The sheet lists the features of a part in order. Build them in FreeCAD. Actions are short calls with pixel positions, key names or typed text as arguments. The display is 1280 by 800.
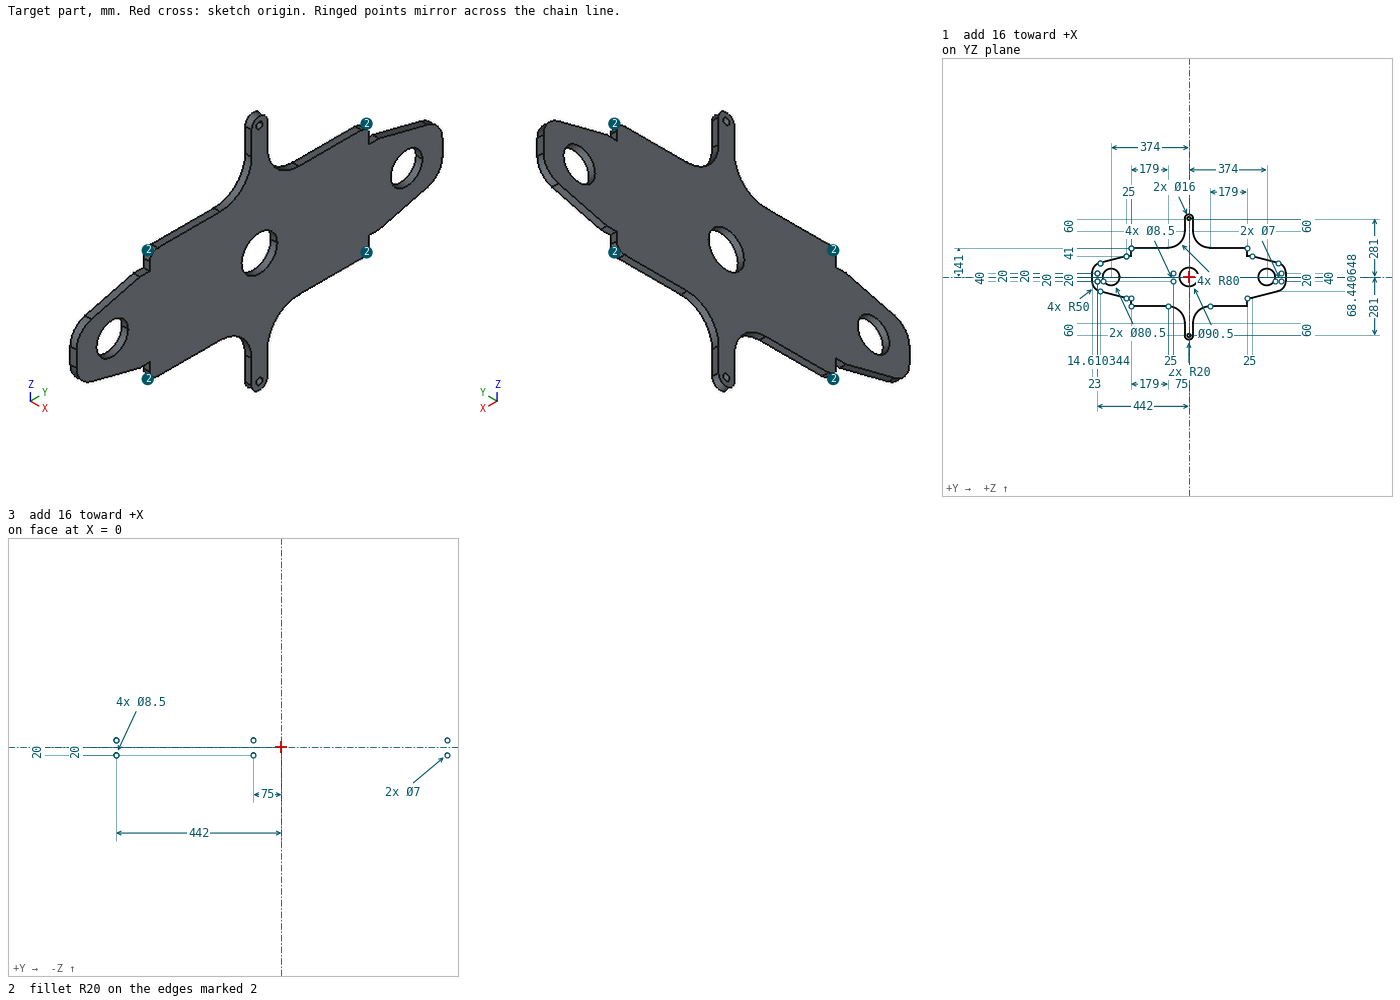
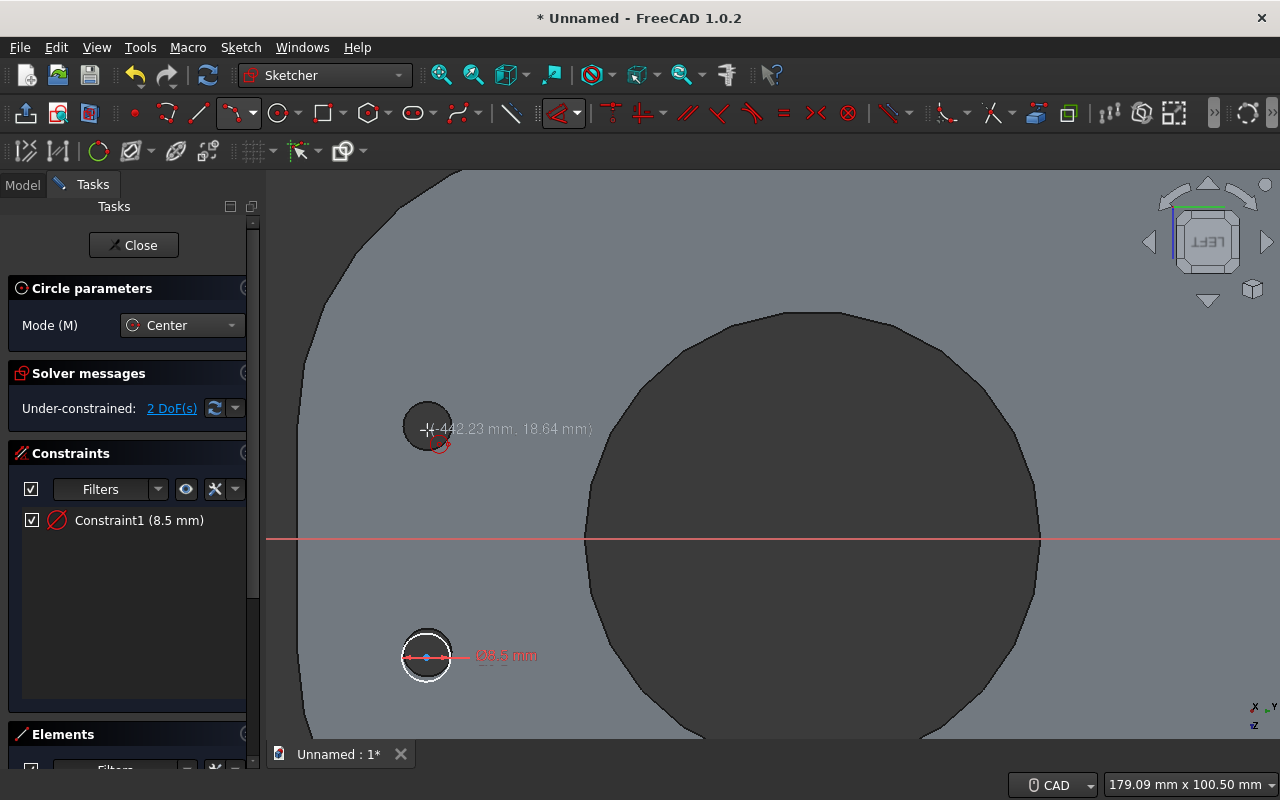
scroll(427, 444, down, 11)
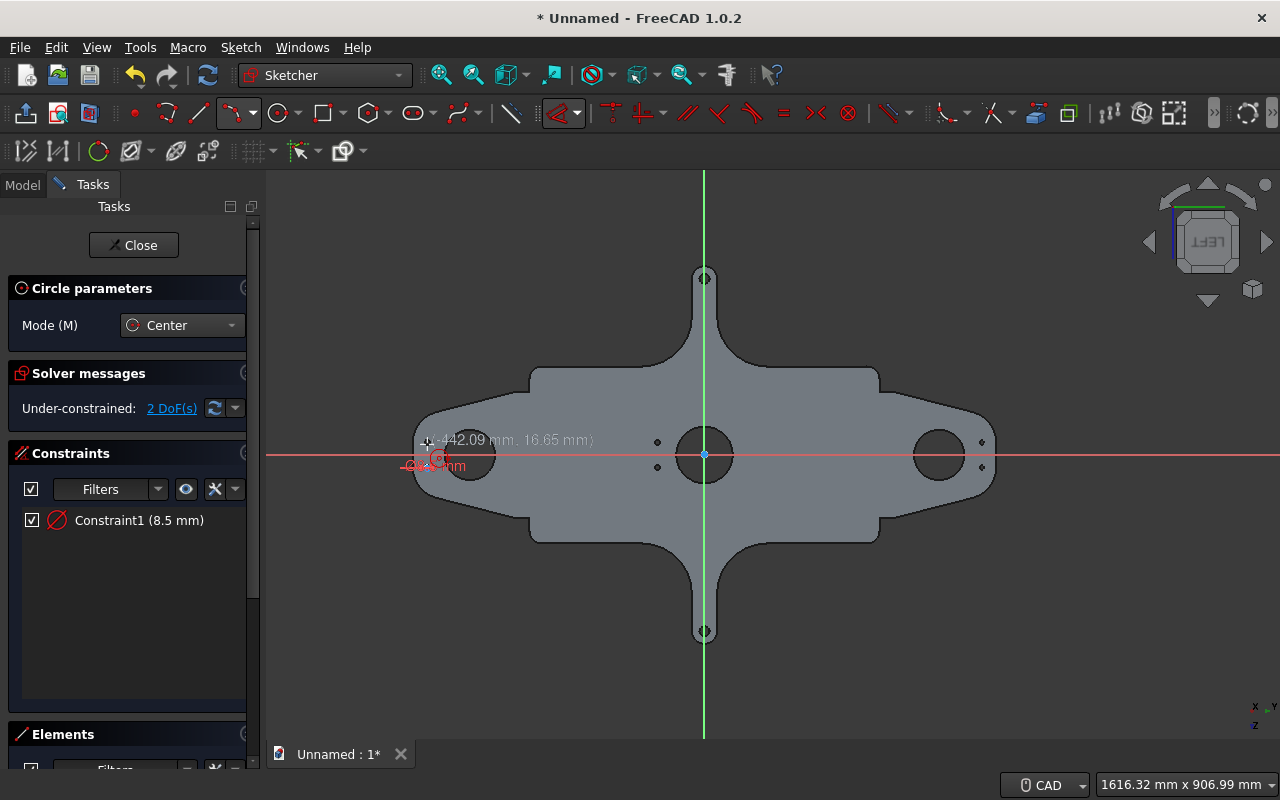
scroll(427, 442, up, 2)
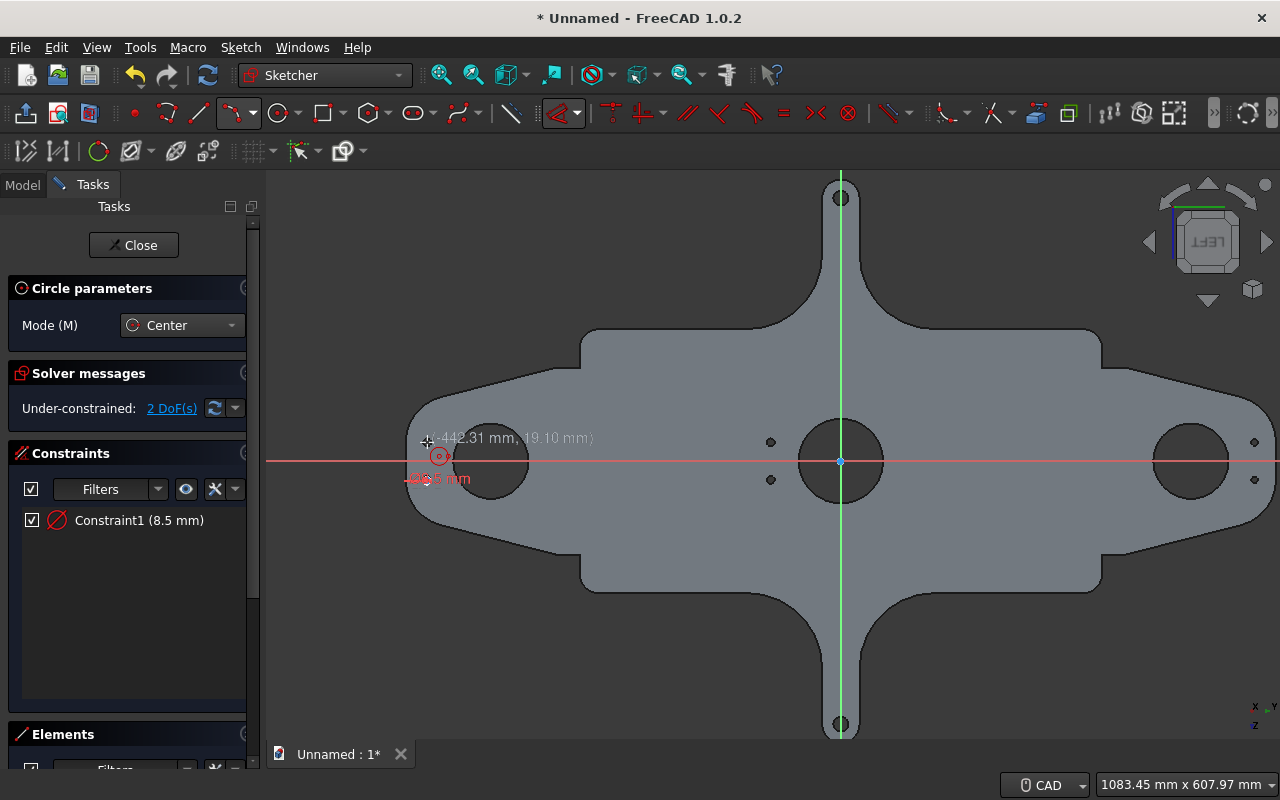
click(427, 442)
move(430, 440)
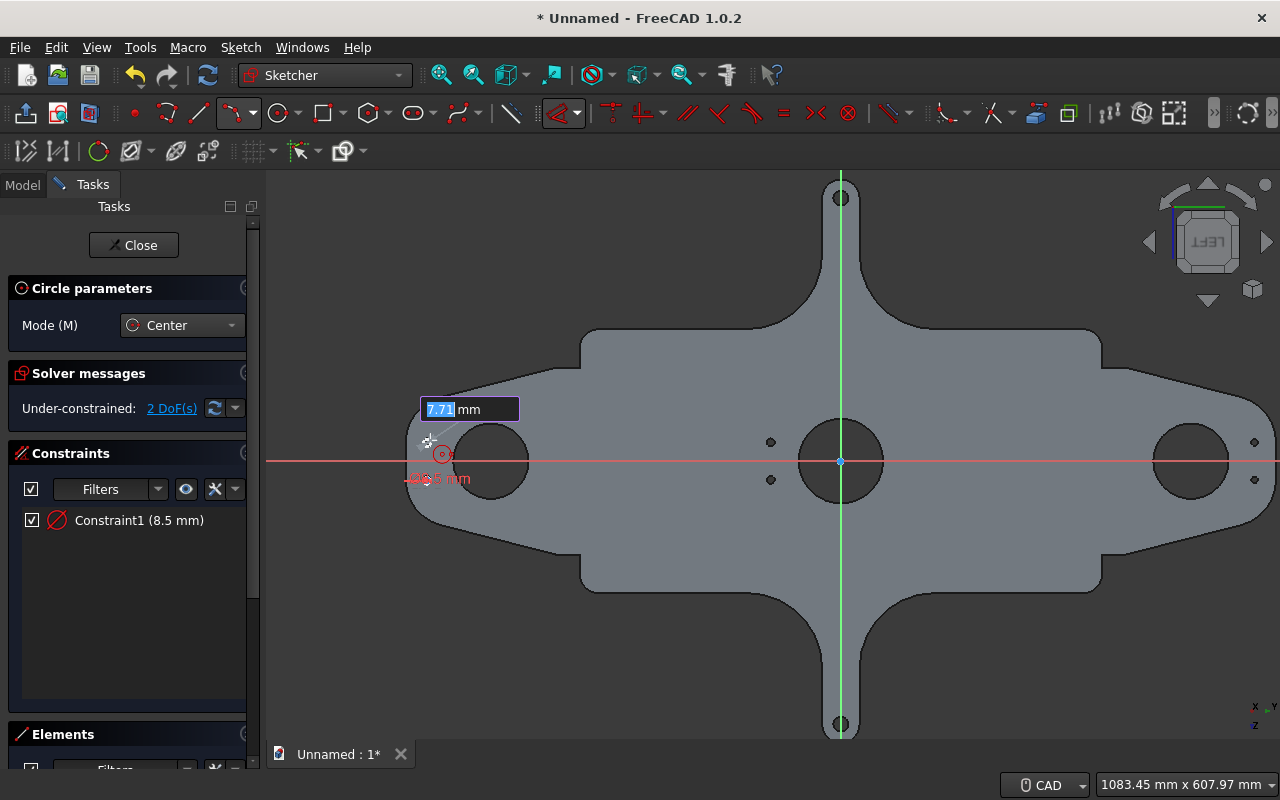
text(8.5)
key(Return)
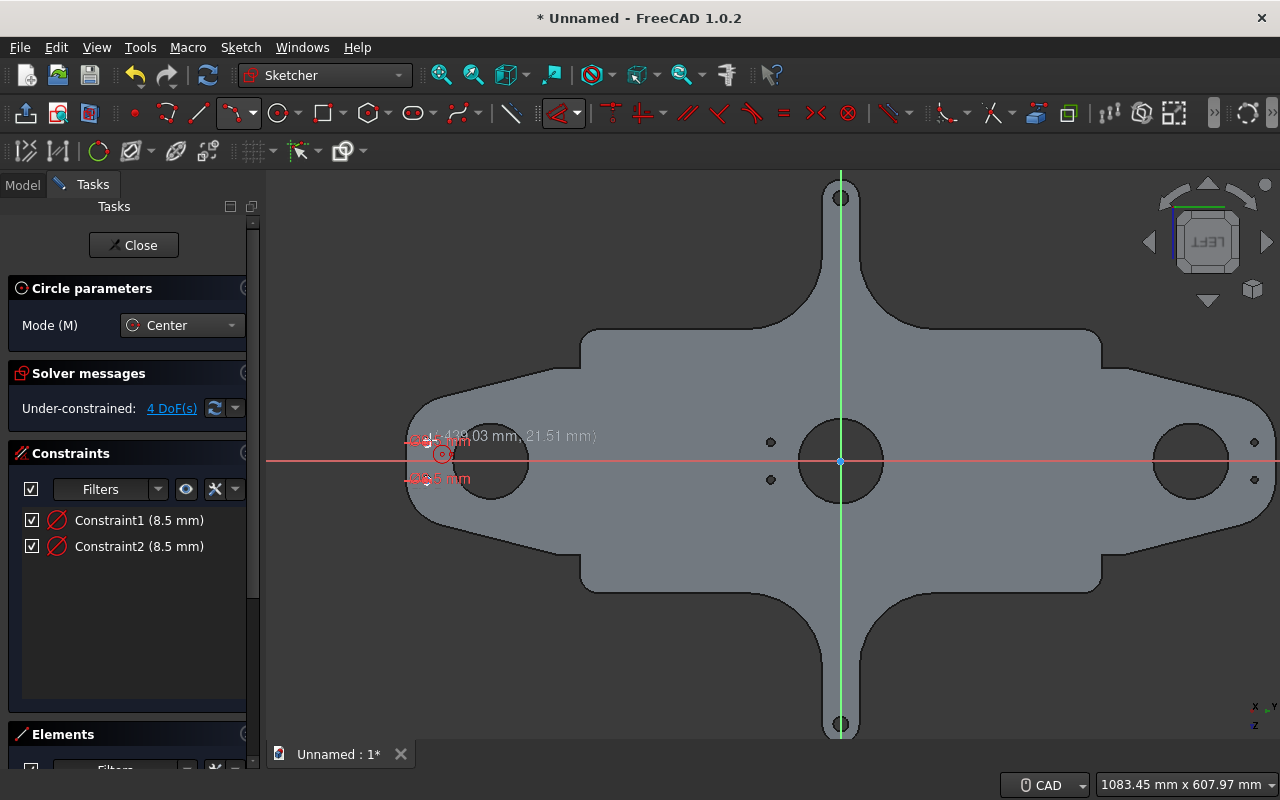
scroll(771, 480, up, 9)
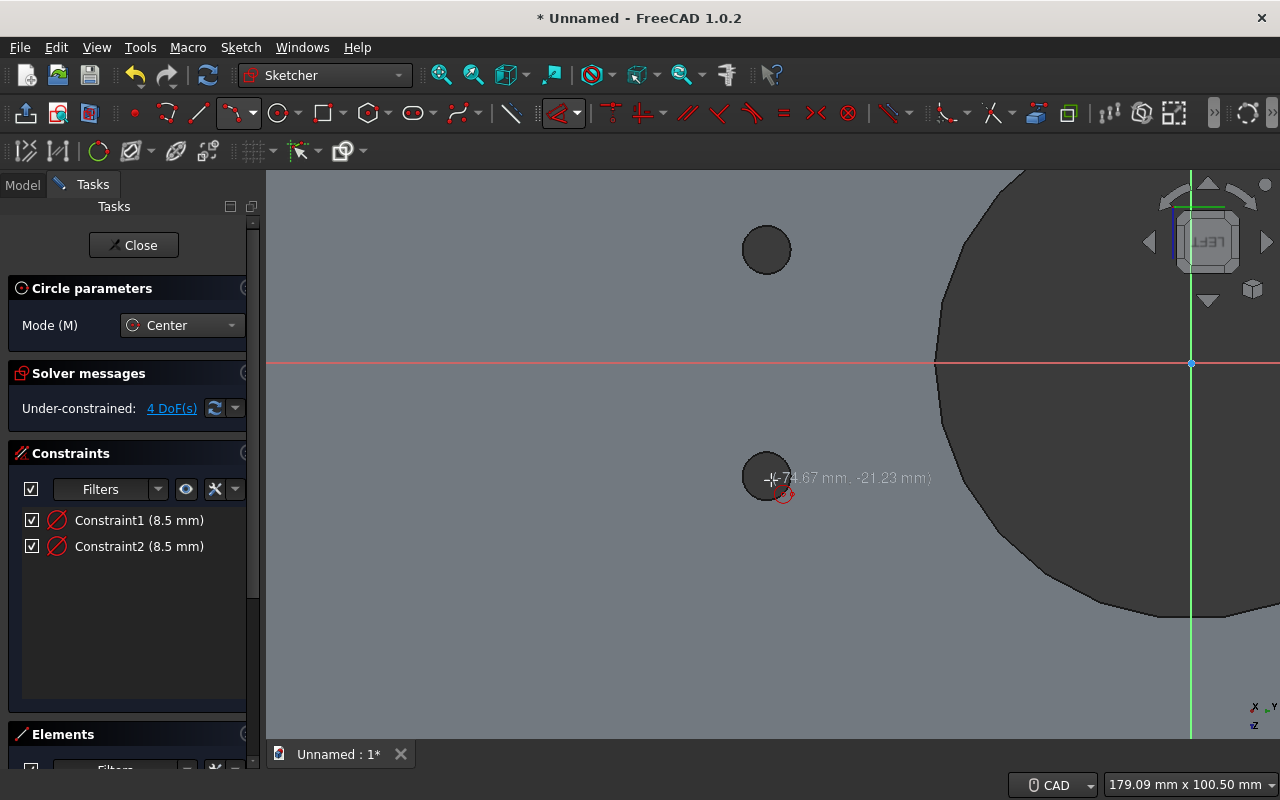
scroll(644, 466, down, 11)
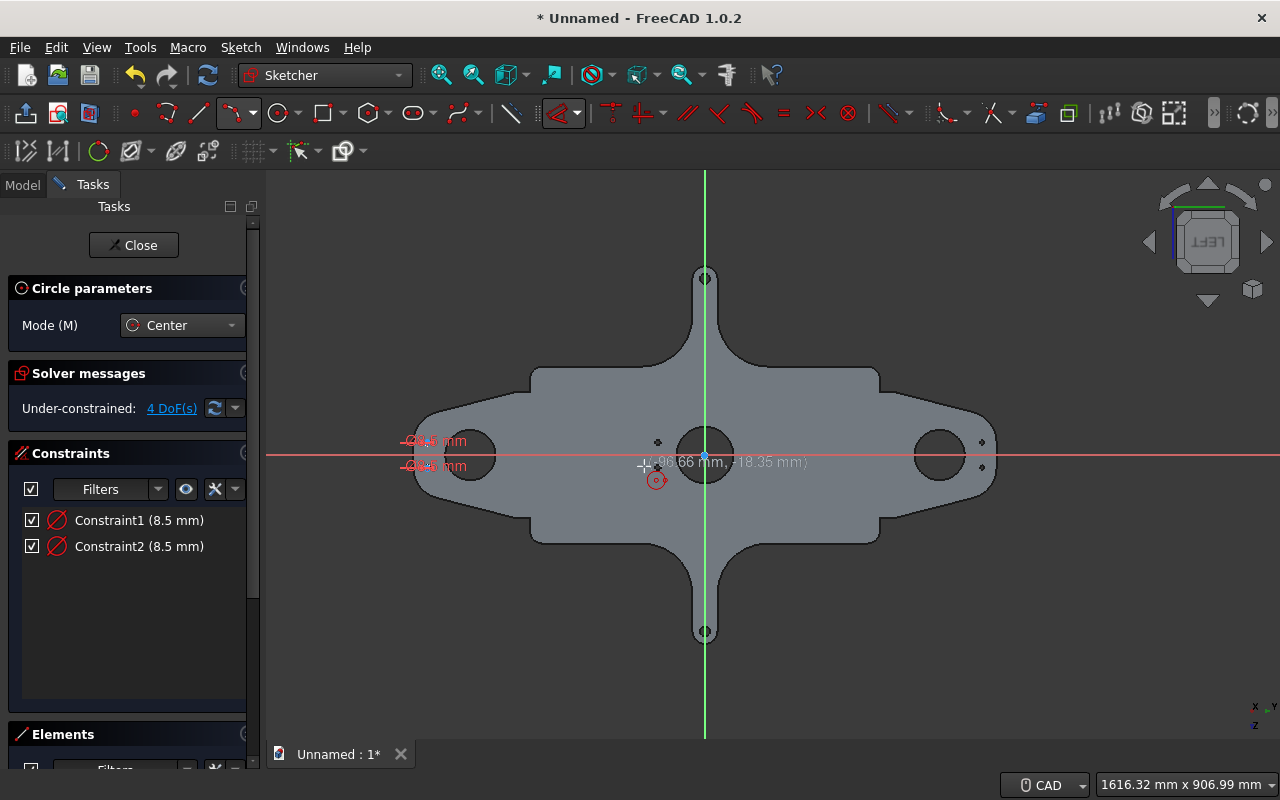
scroll(658, 468, up, 2)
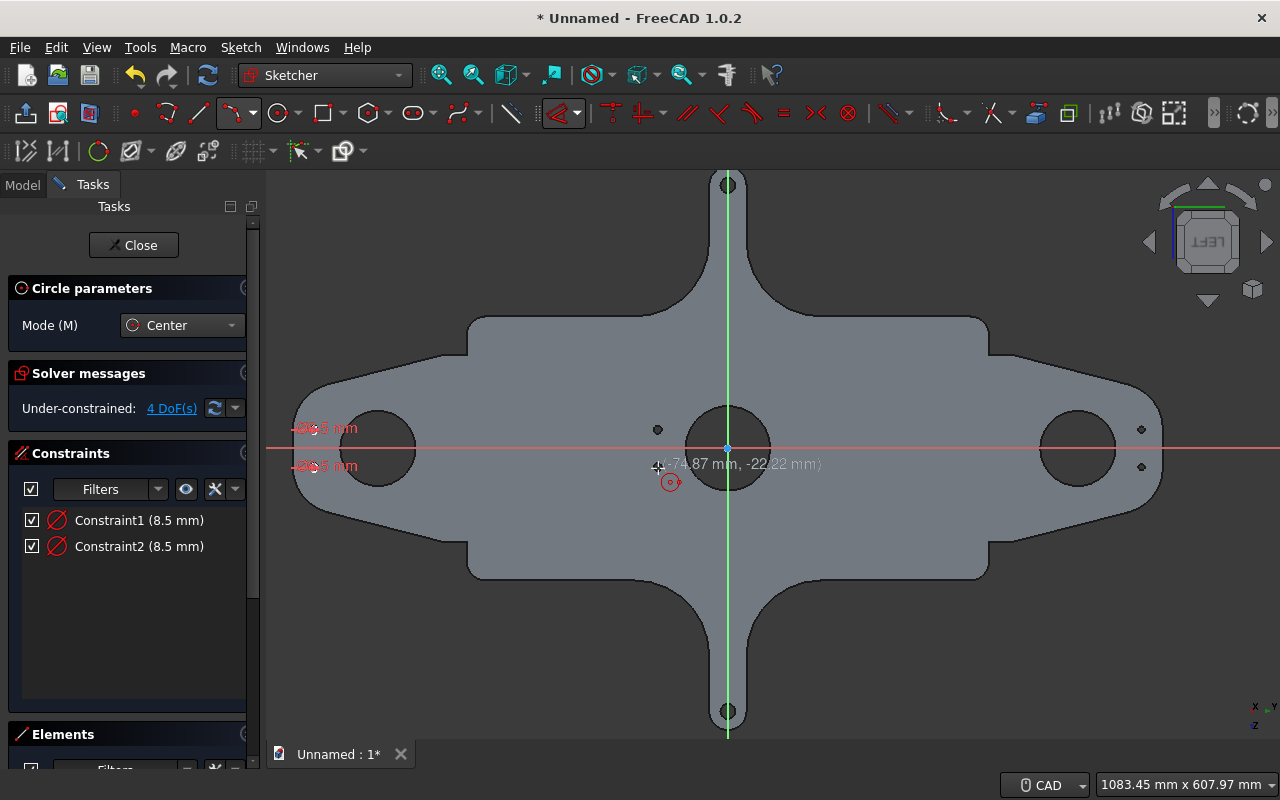
click(658, 467)
move(660, 464)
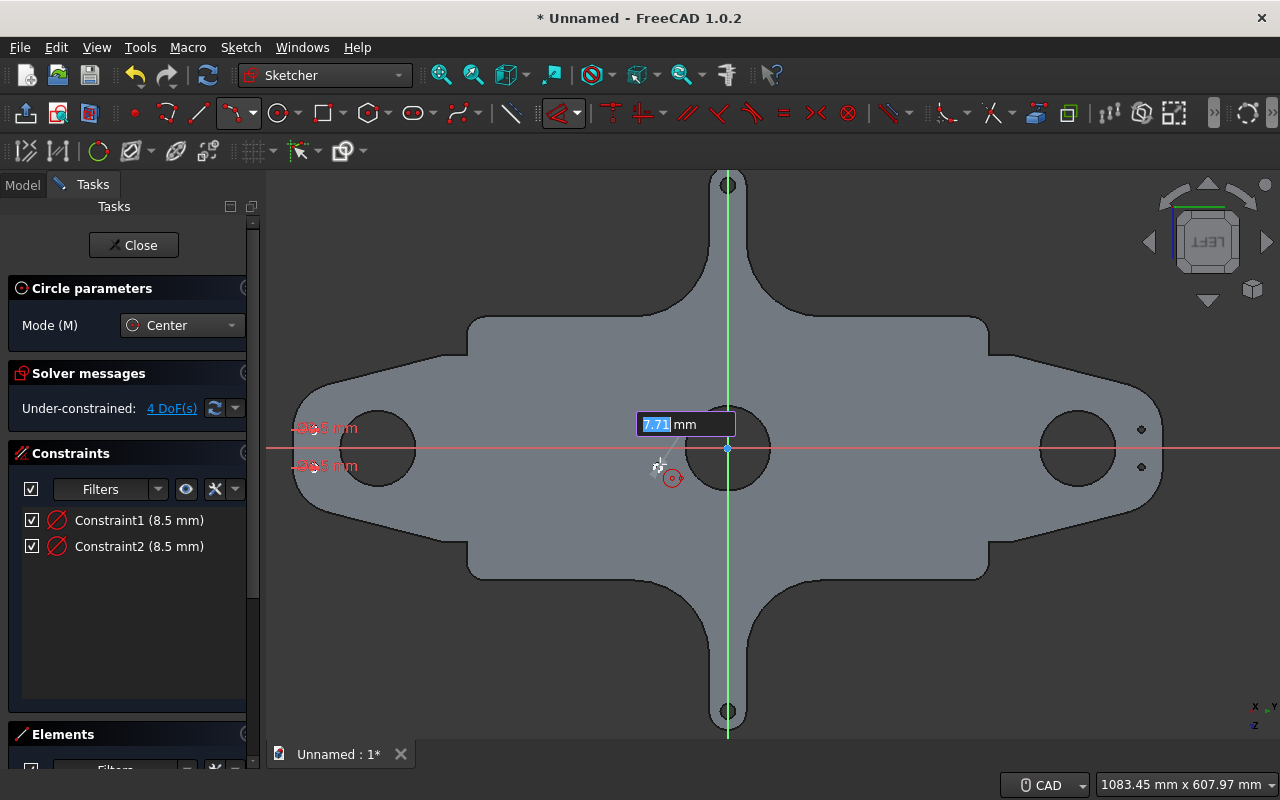
text(8.5)
key(Return)